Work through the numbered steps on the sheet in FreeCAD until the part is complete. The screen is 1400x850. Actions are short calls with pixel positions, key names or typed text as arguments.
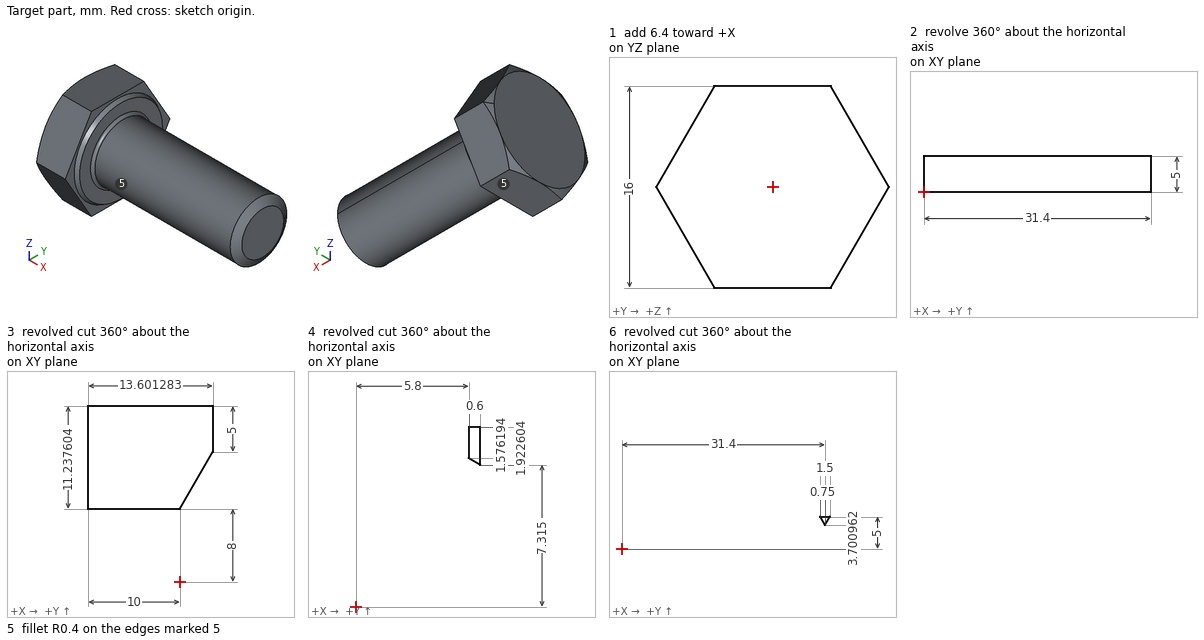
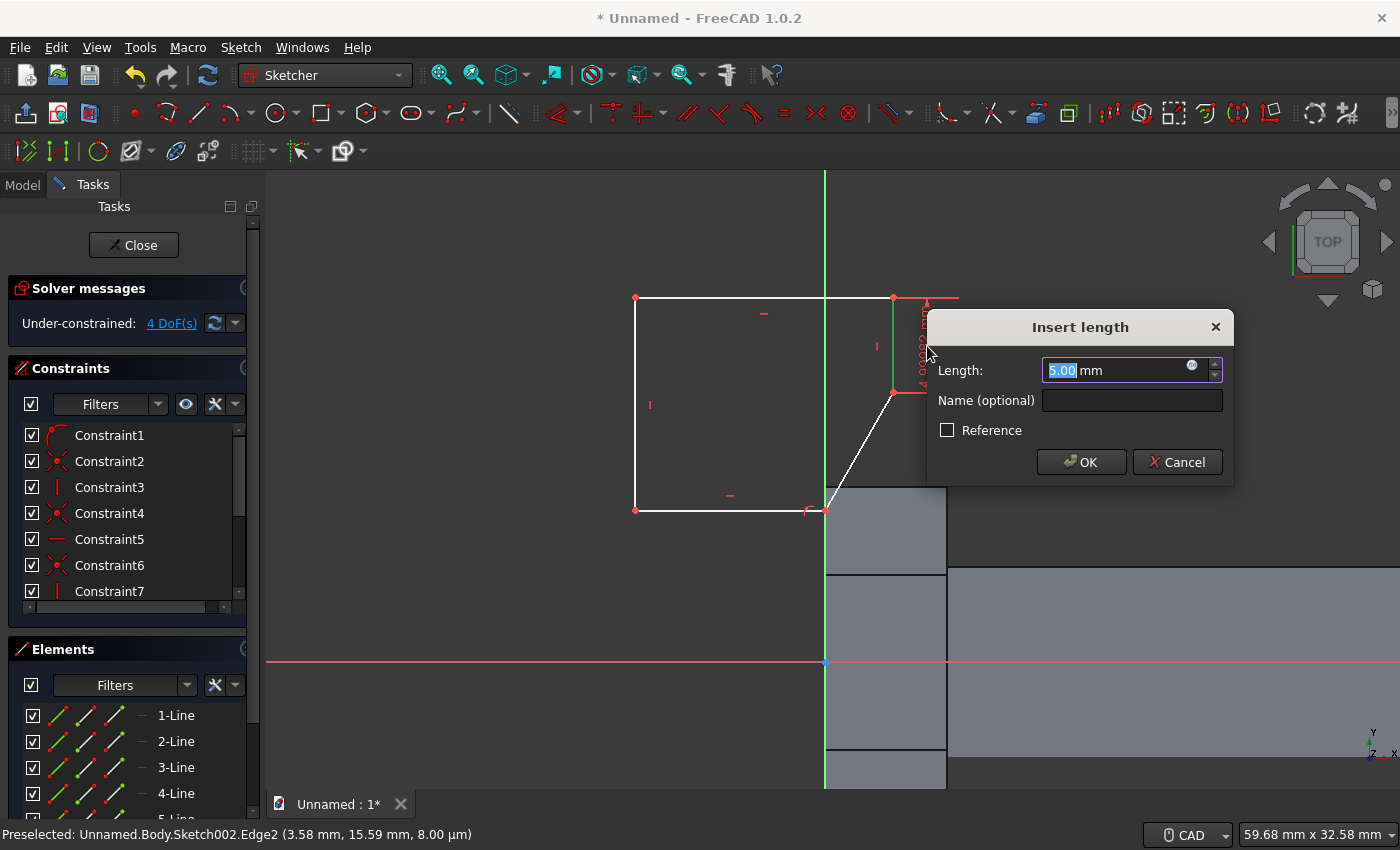
text(5)
key(Return)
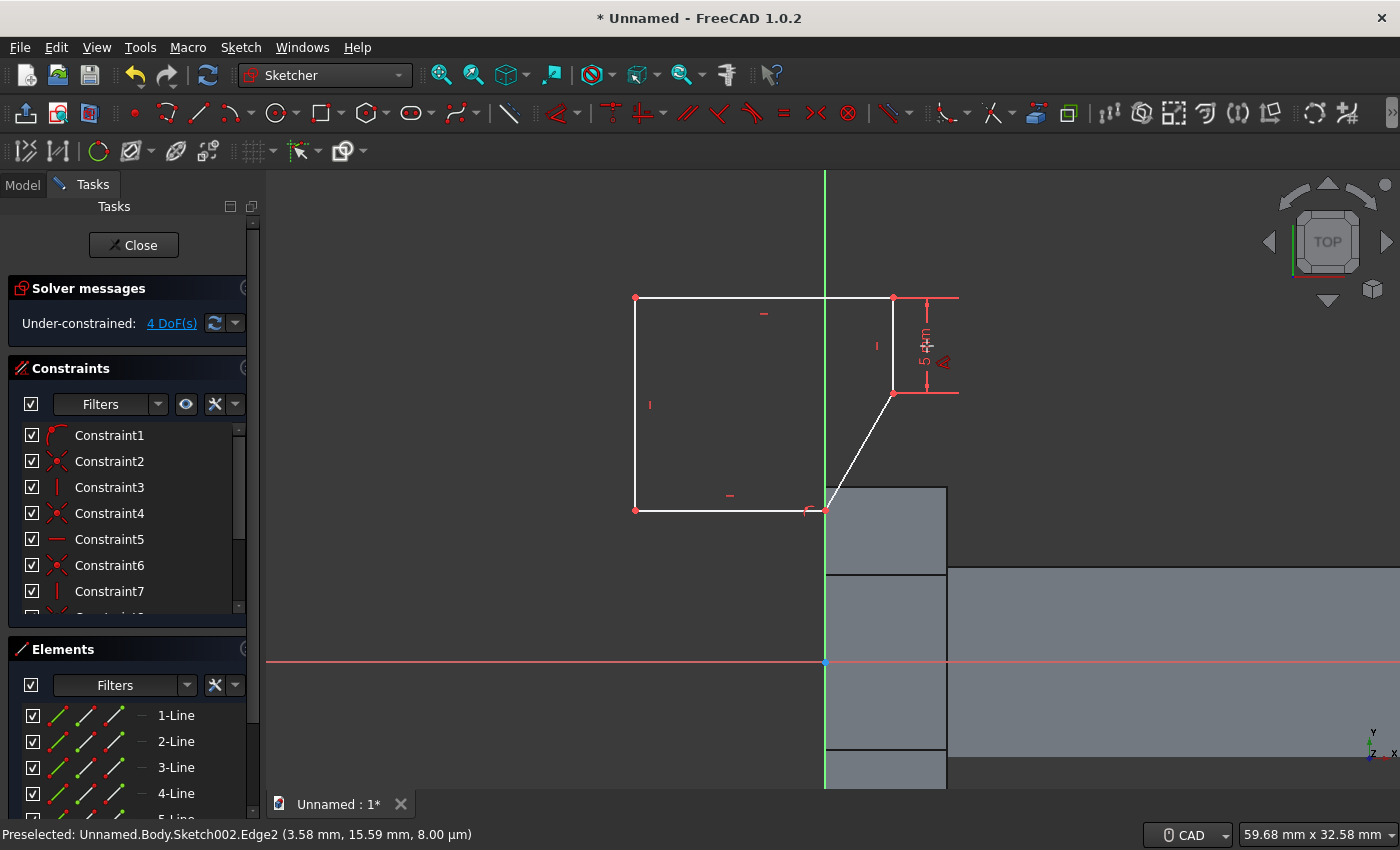
click(692, 511)
click(730, 545)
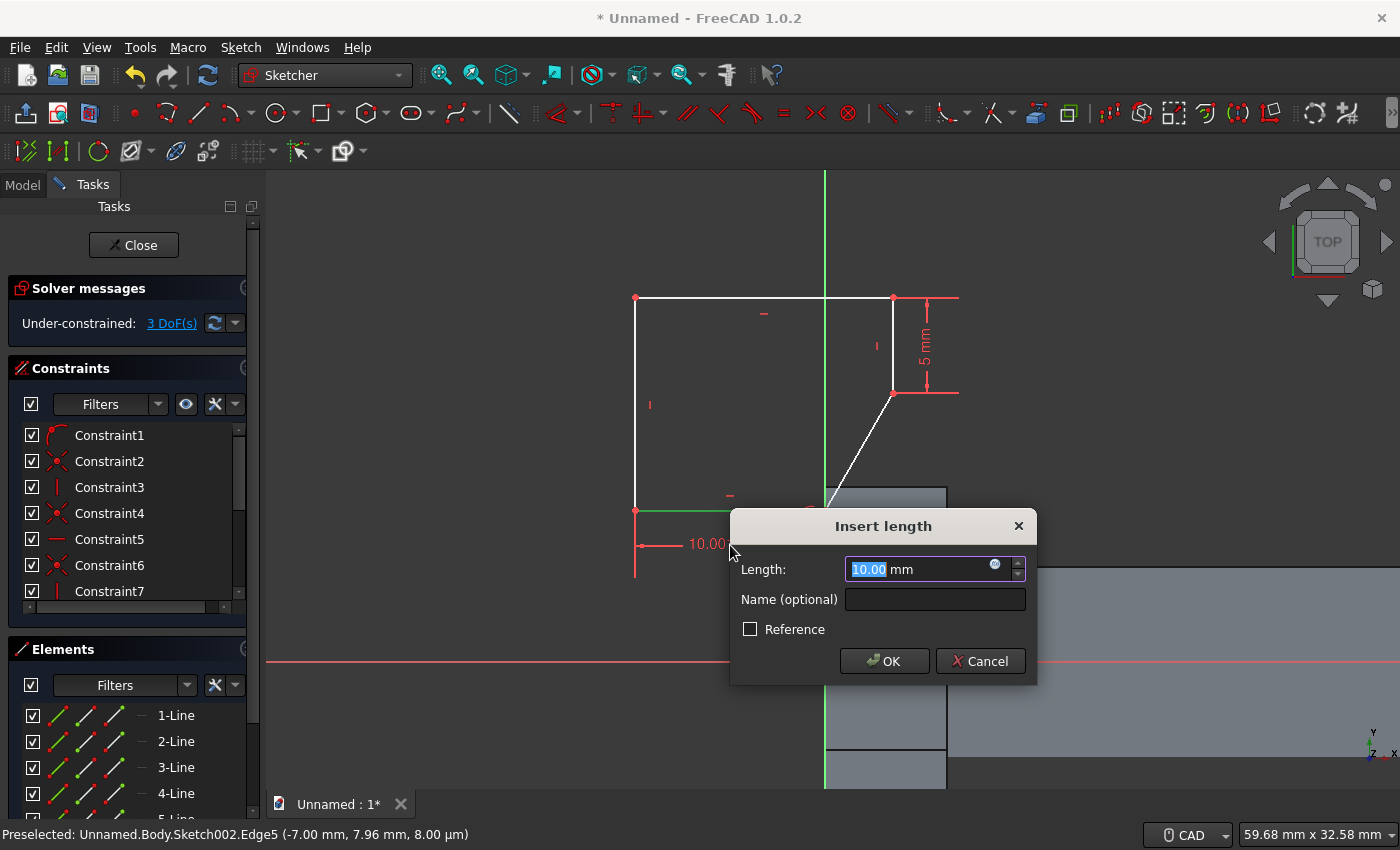
text(10)
key(Return)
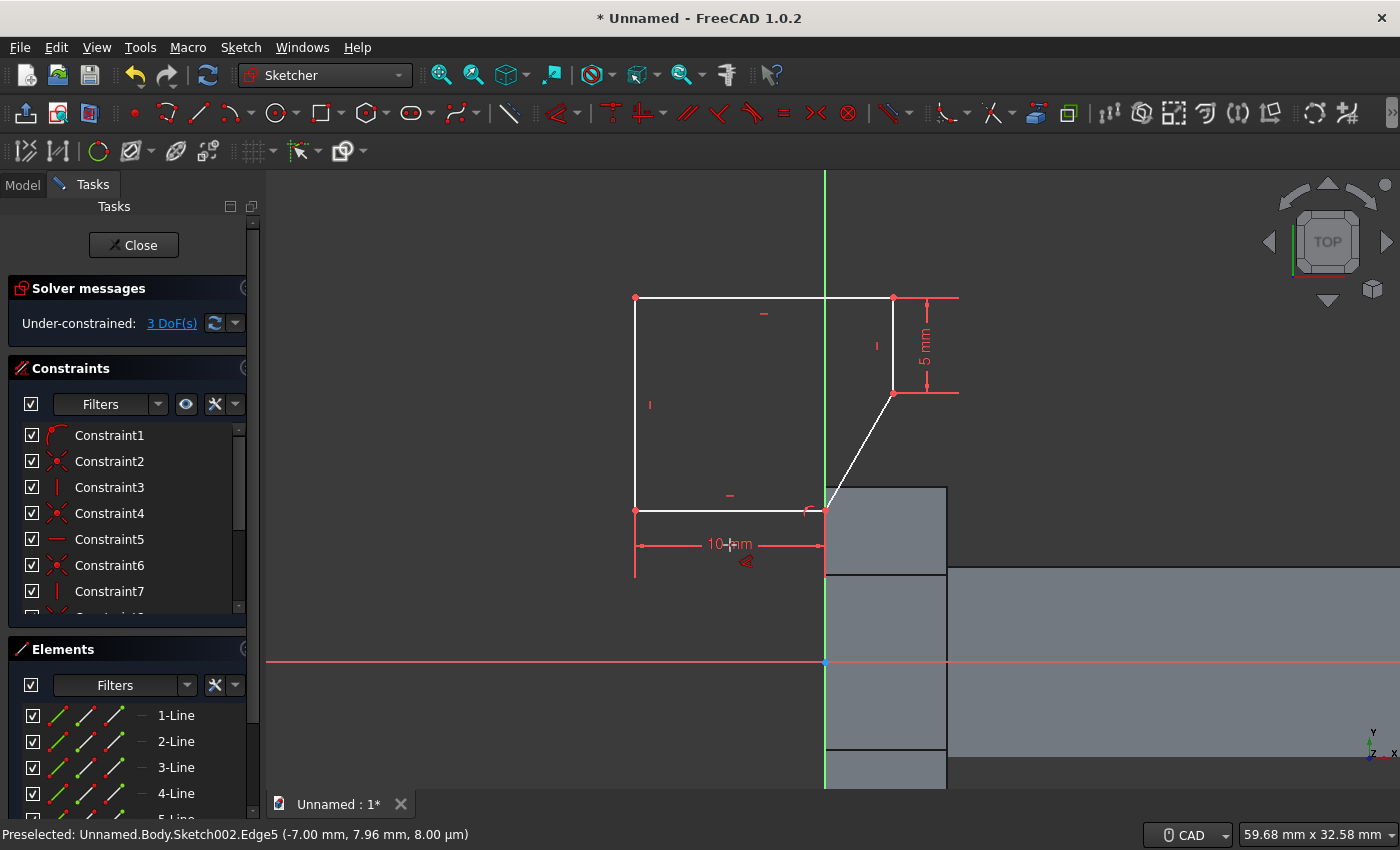
click(825, 511)
click(859, 587)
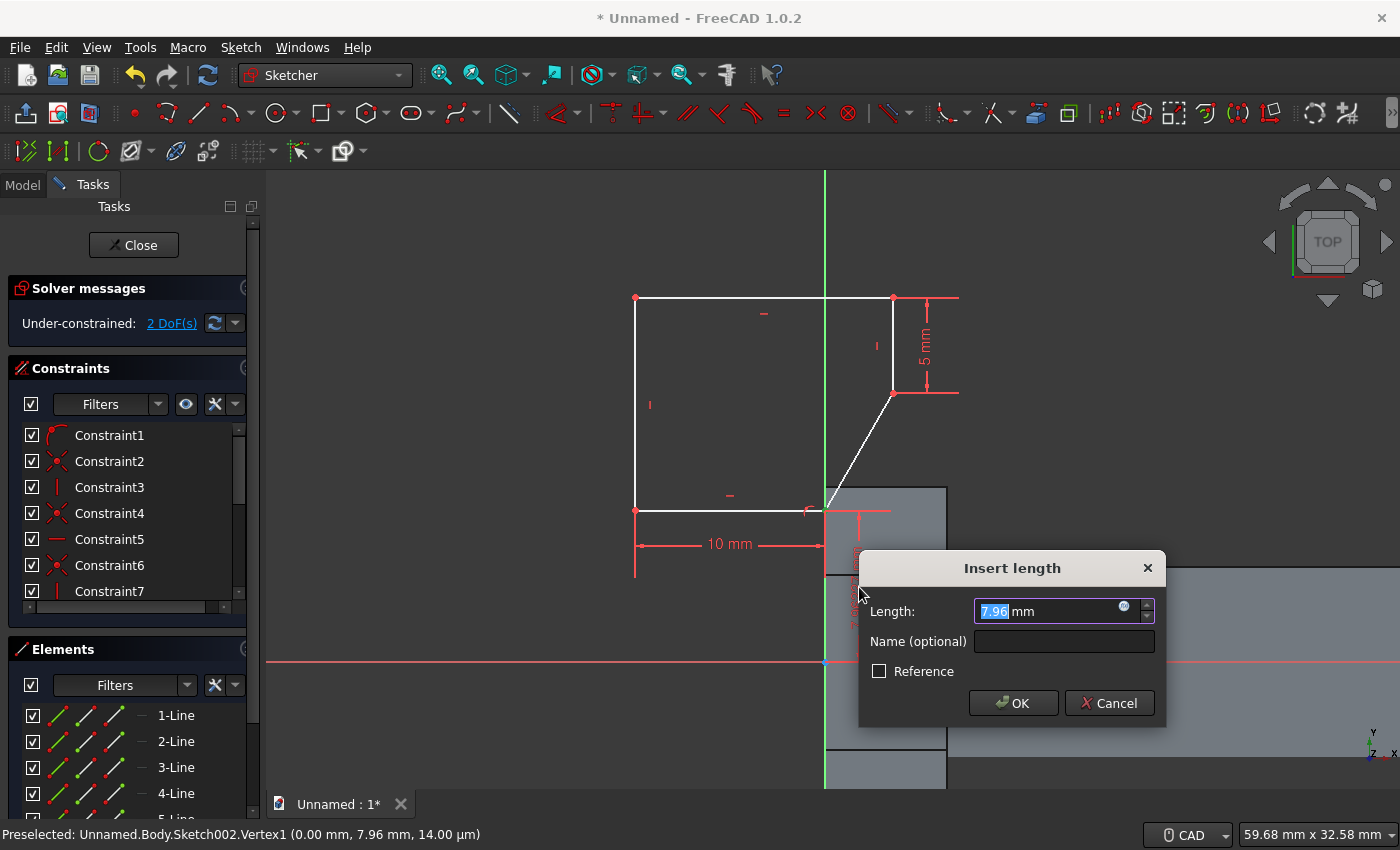
text(8)
key(Return)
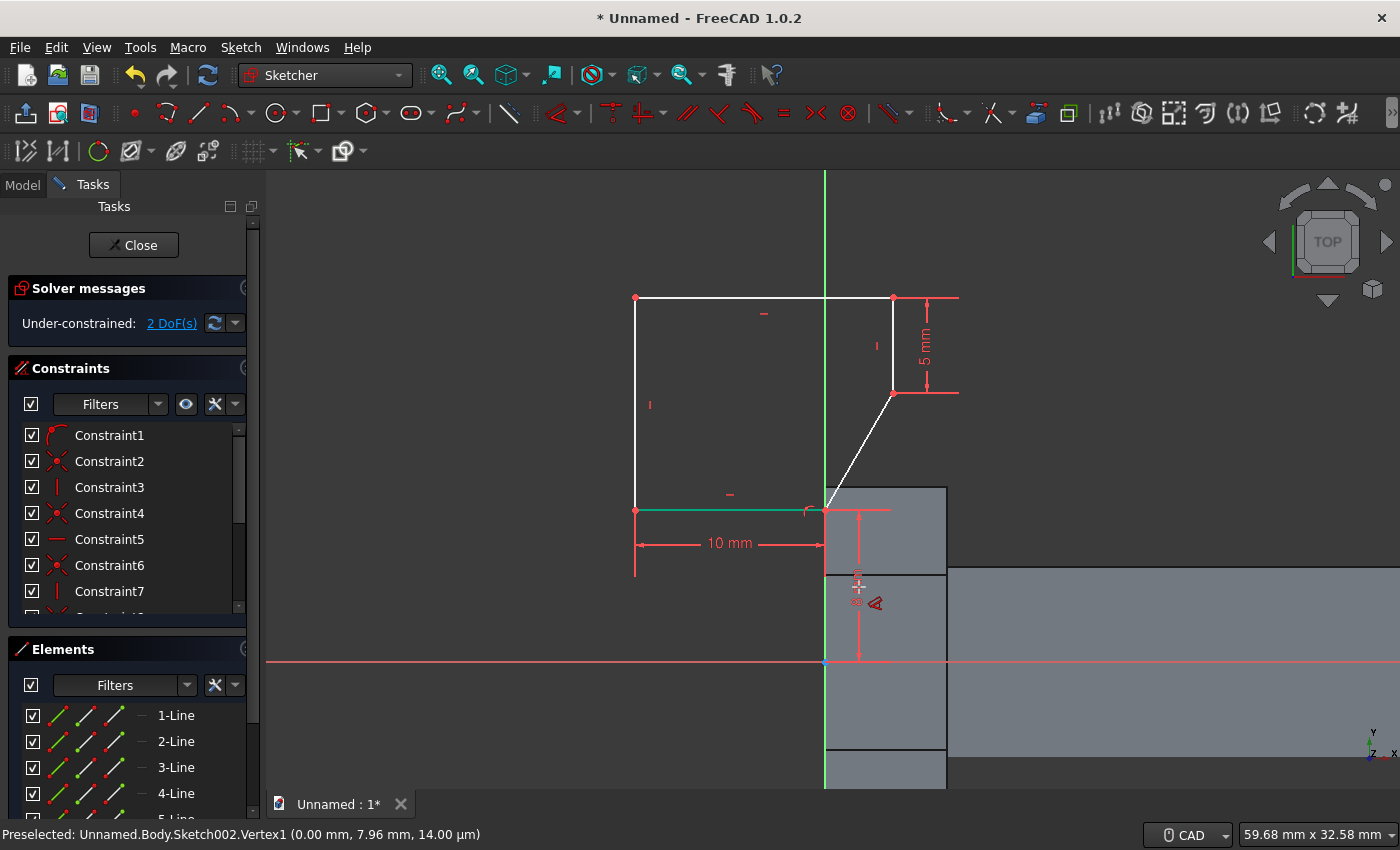
scroll(816, 298, up, 2)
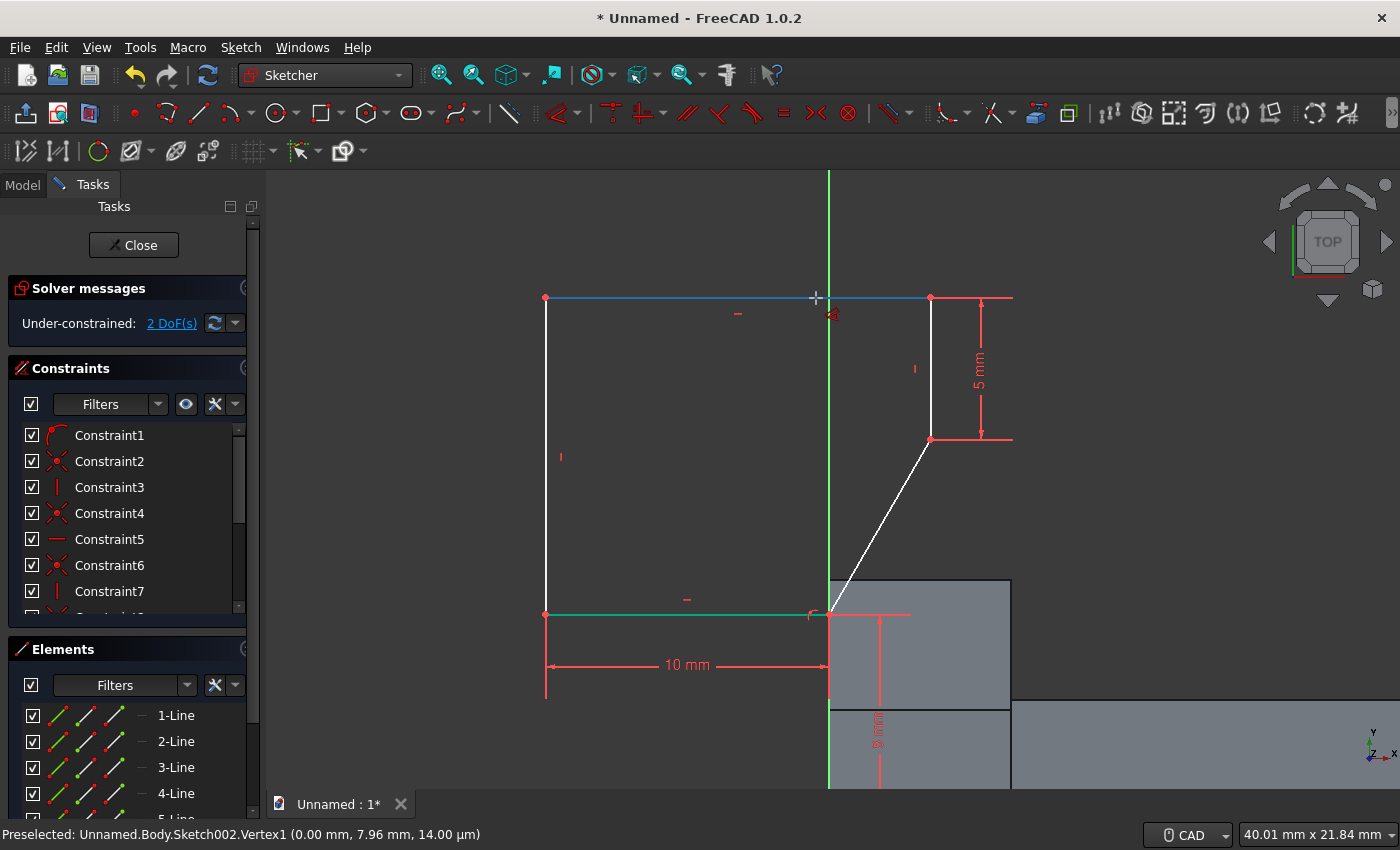
click(815, 298)
click(738, 264)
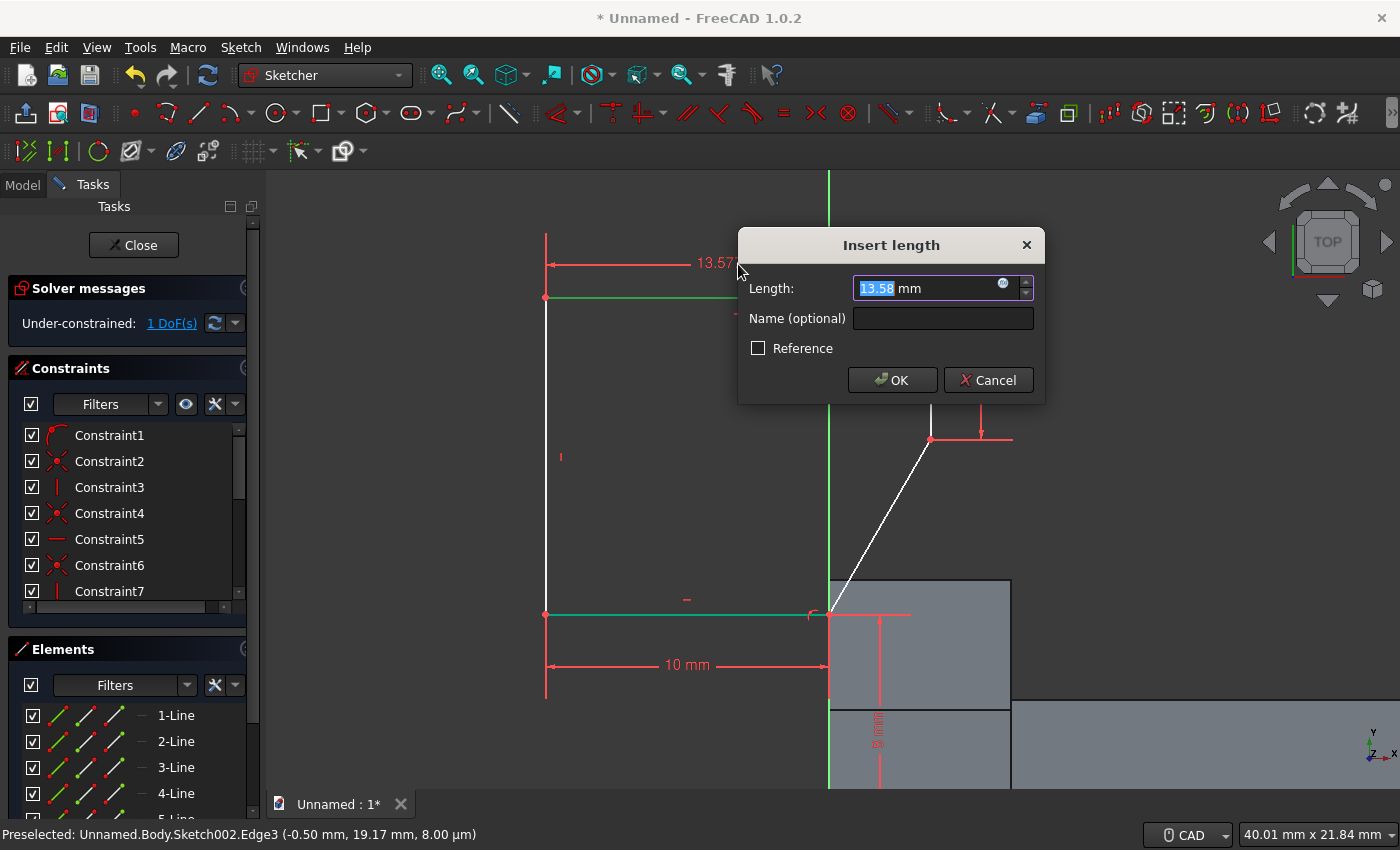
text(13.601283)
key(Return)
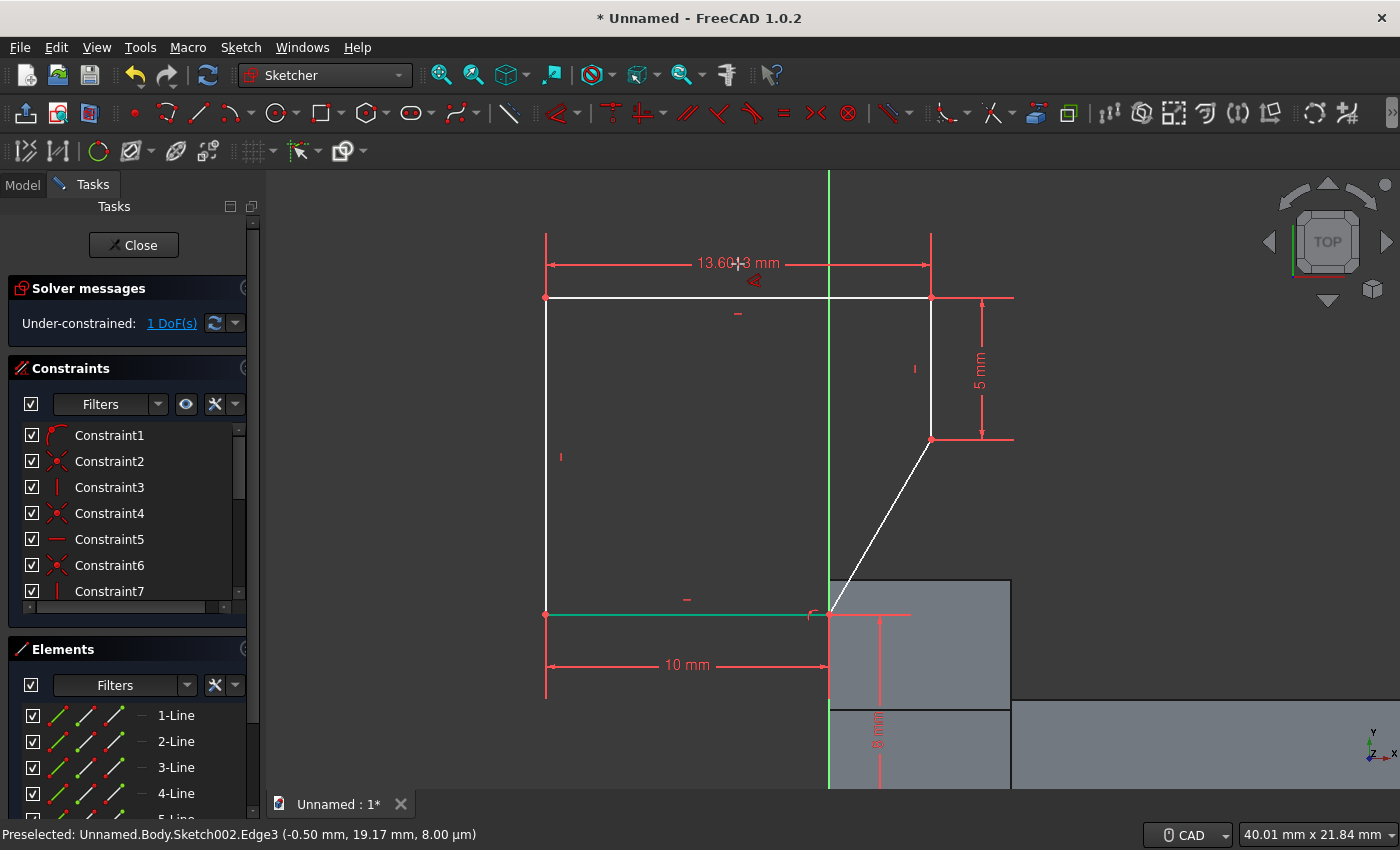
click(546, 393)
click(512, 456)